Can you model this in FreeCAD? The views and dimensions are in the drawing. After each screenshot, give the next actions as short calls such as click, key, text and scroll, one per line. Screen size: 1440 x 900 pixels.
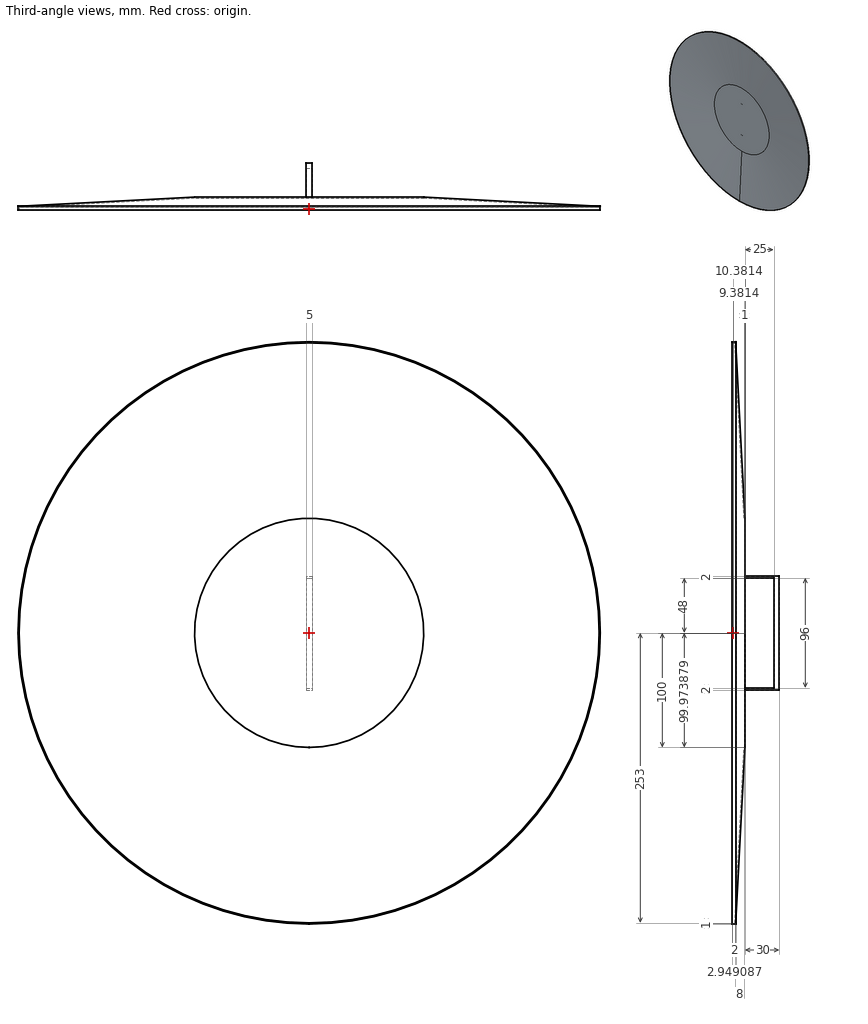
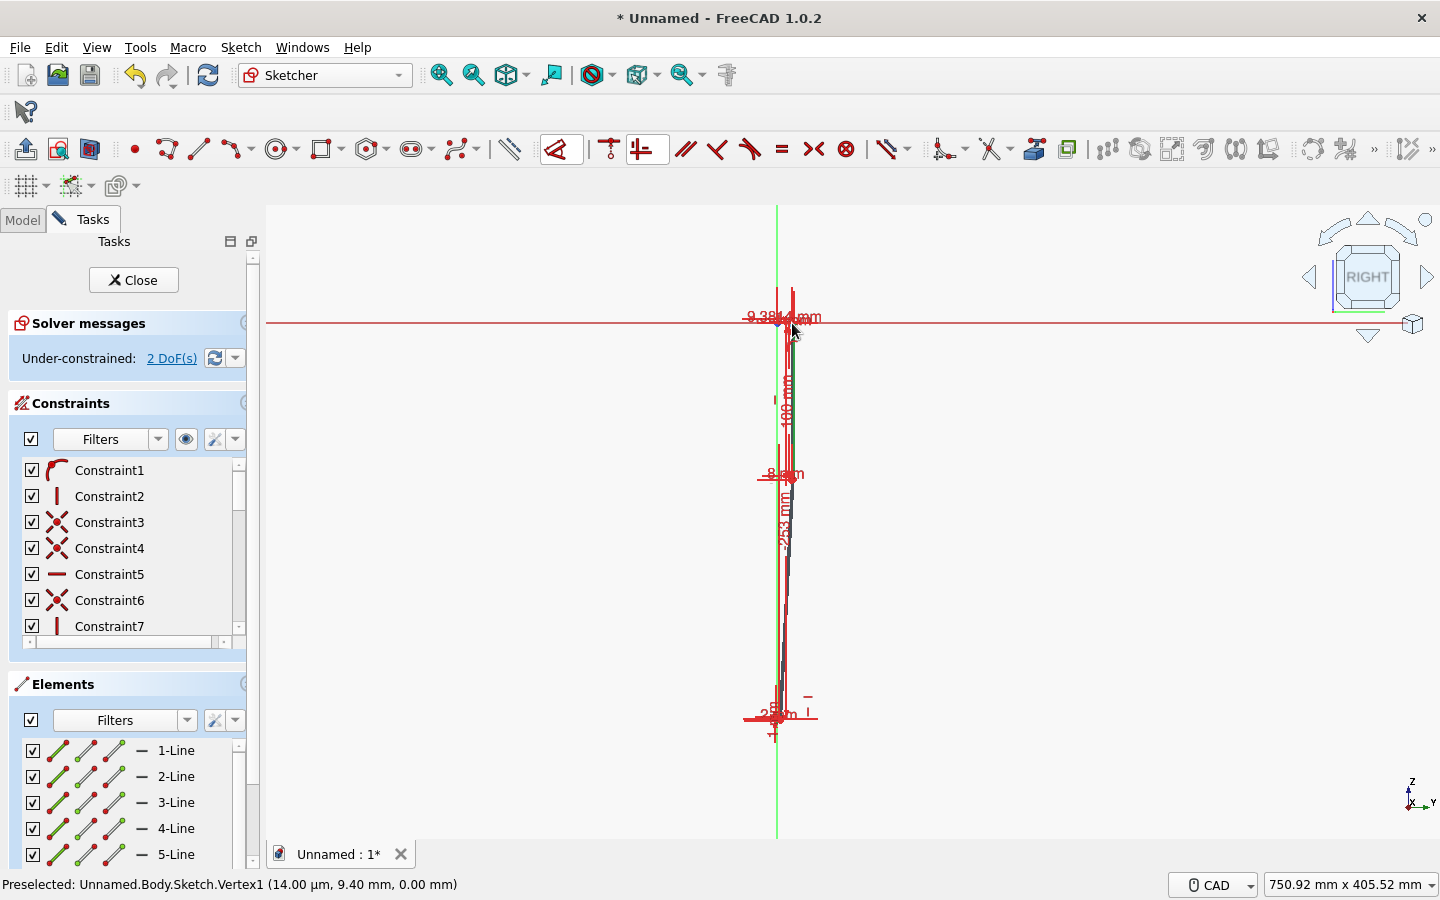
scroll(778, 721, up, 12)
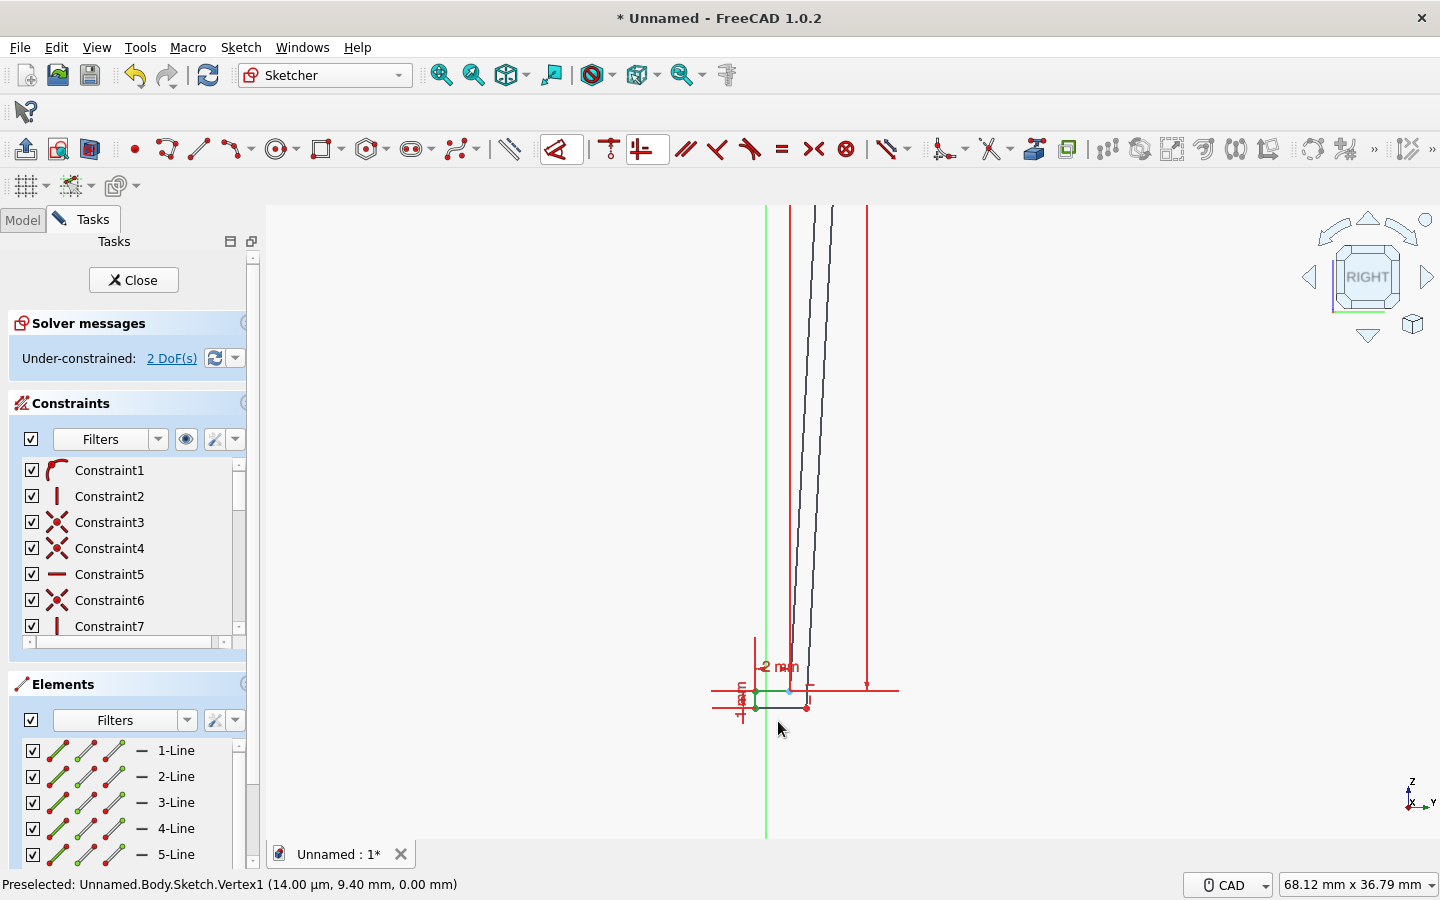
click(771, 708)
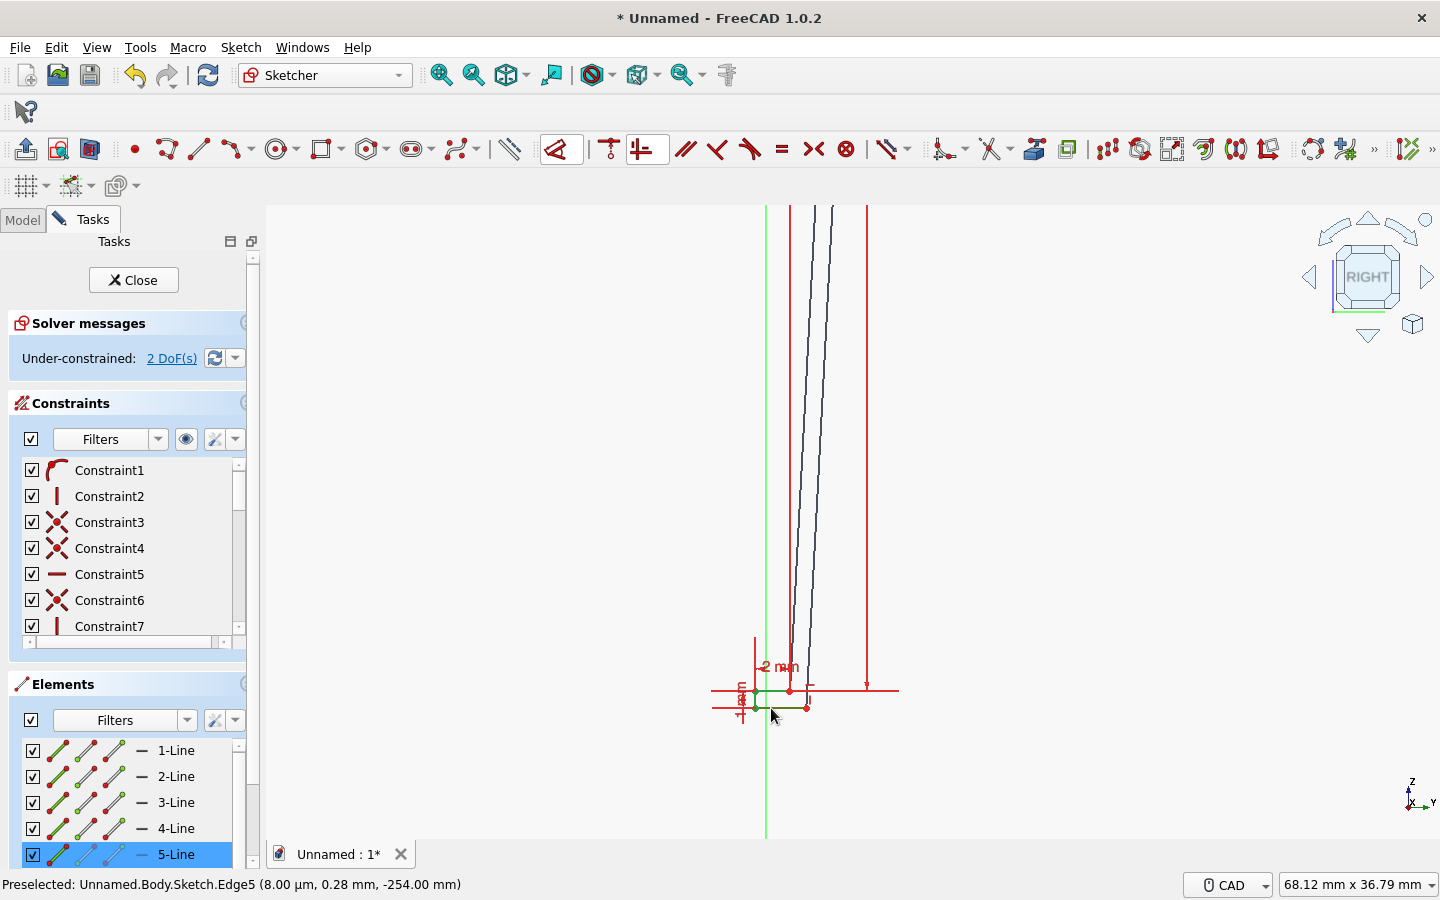
key(l)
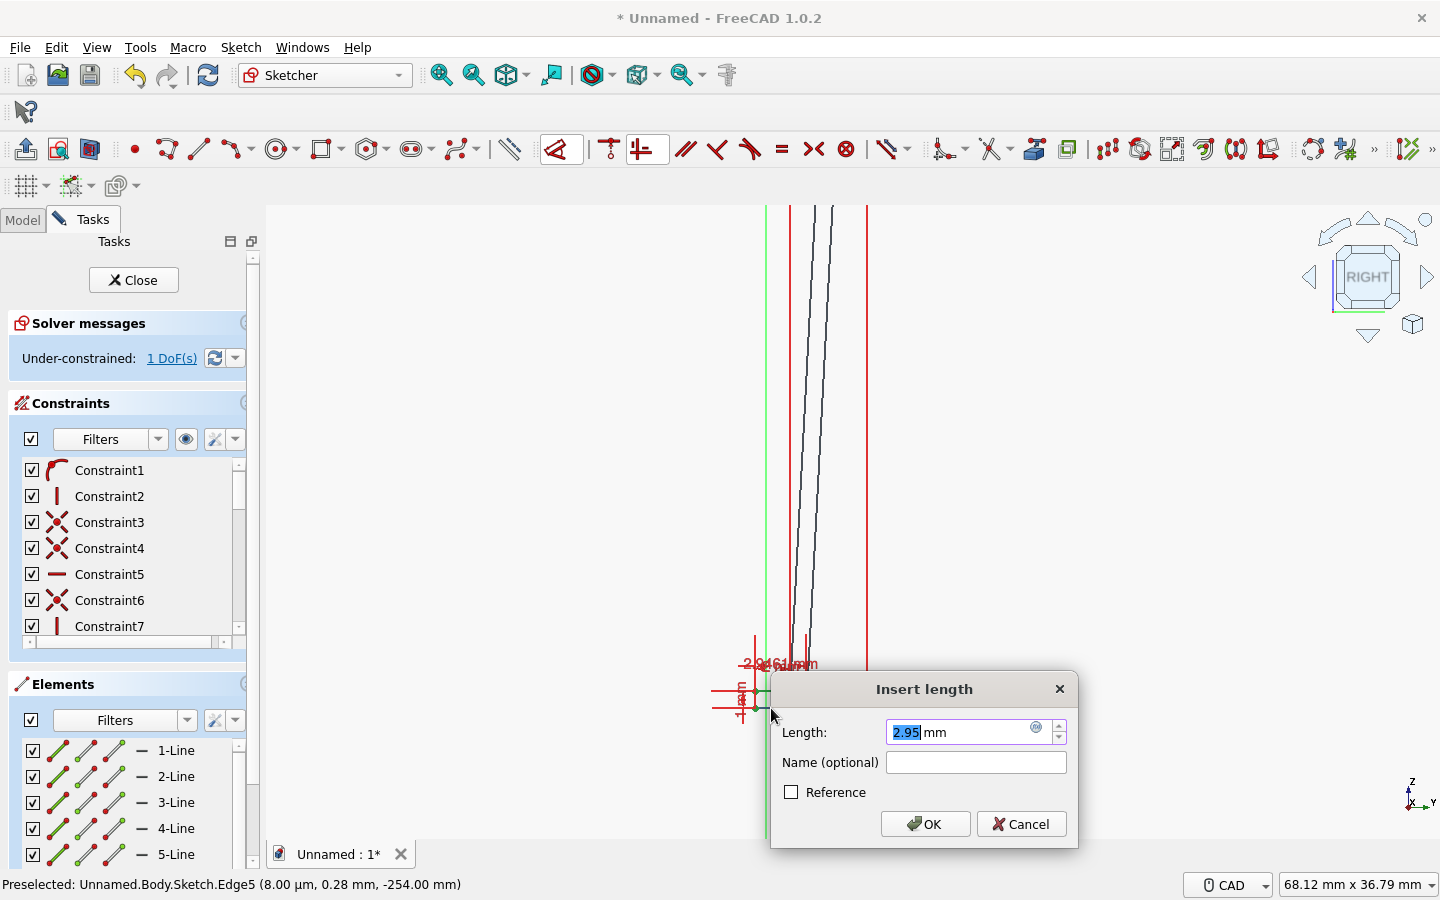
text(2.949087)
key(Return)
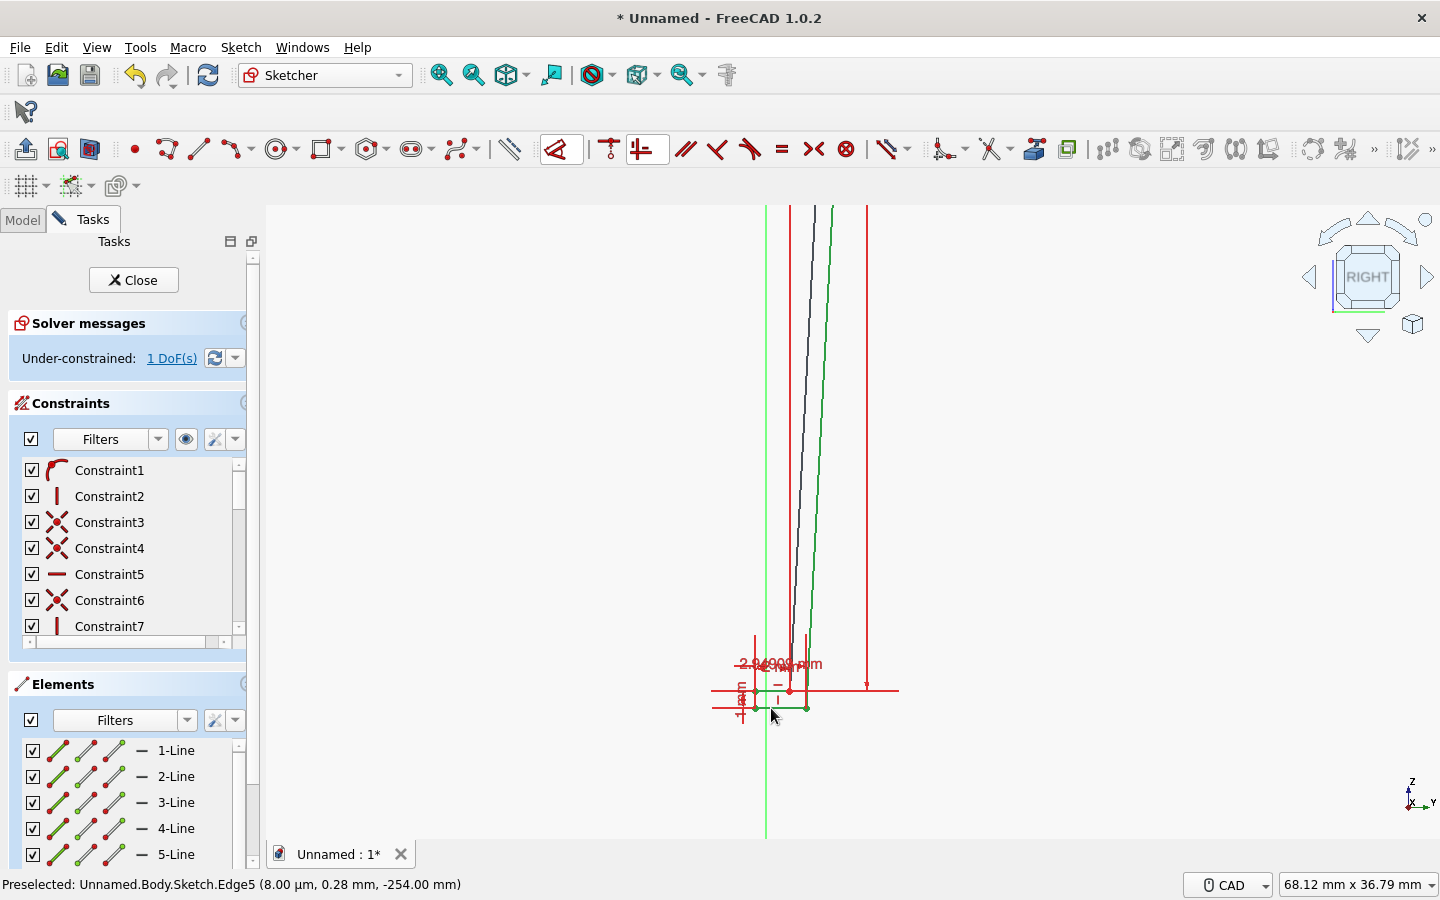
scroll(778, 722, down, 12)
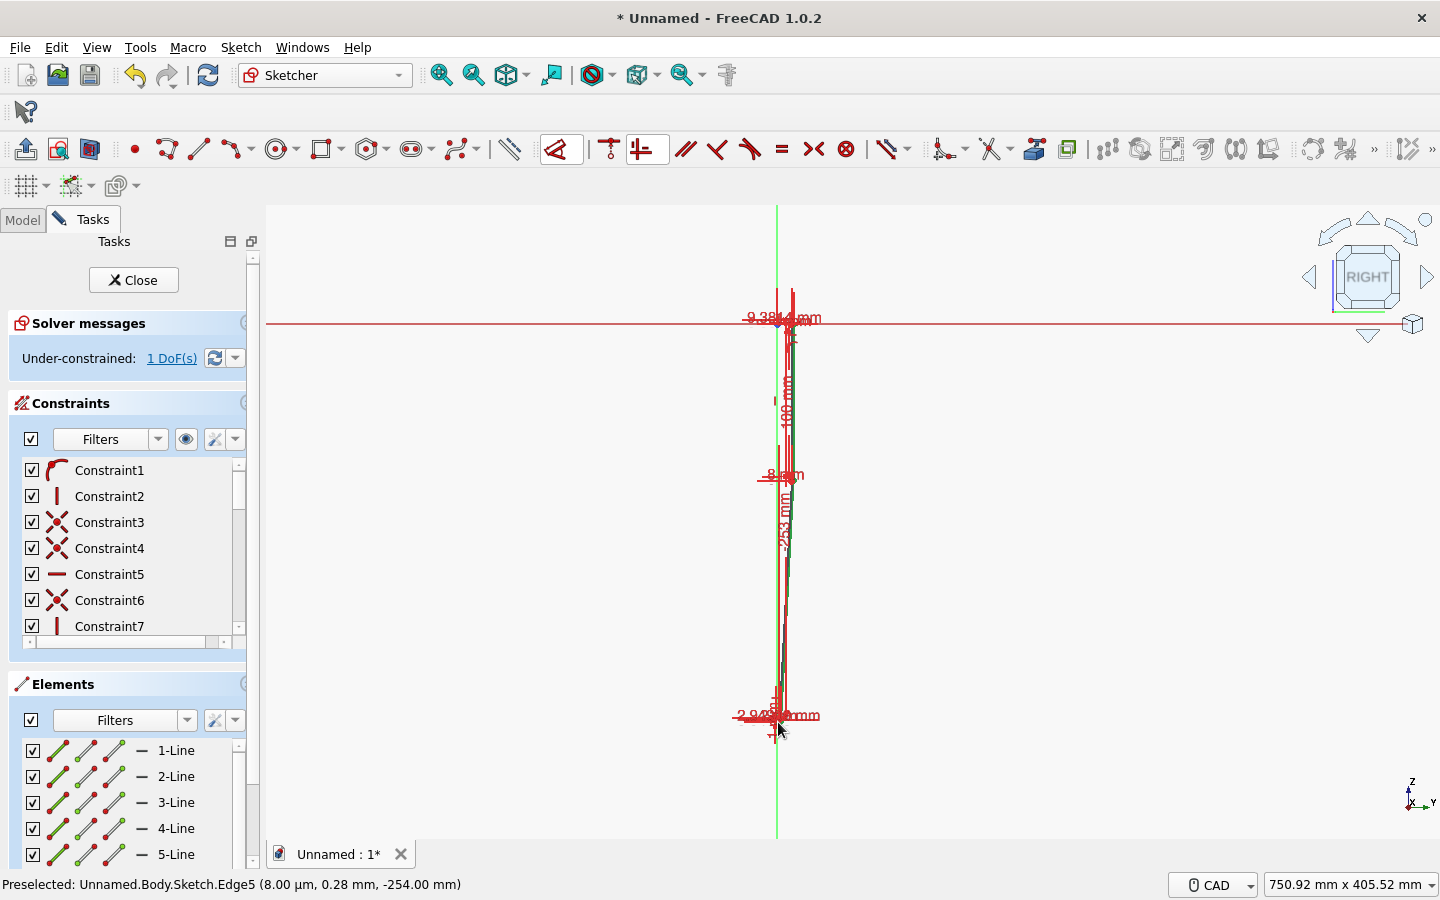
scroll(792, 371, up, 11)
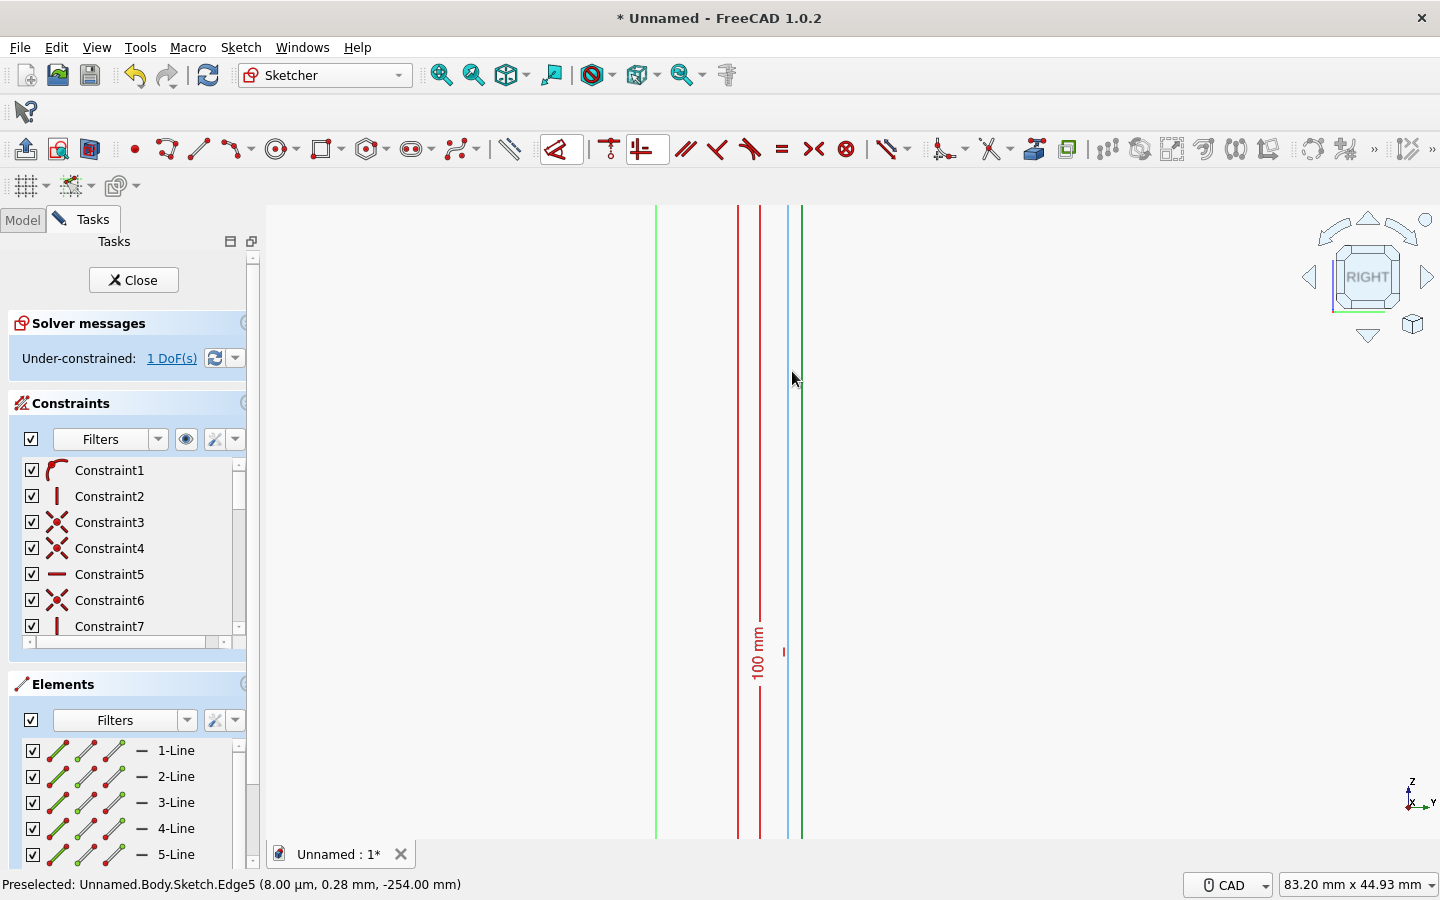
click(788, 373)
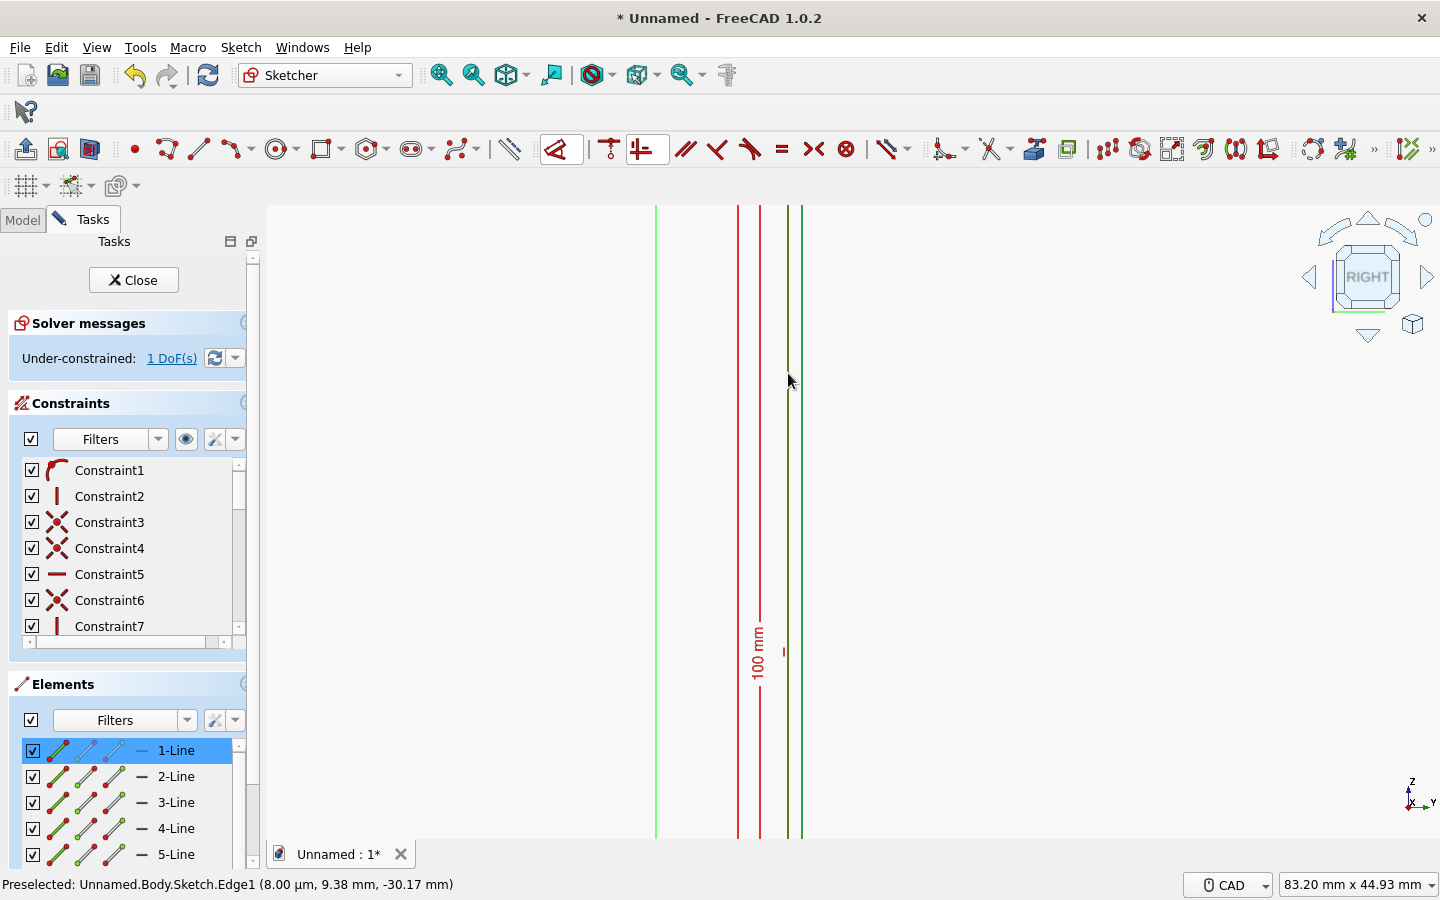
key(i)